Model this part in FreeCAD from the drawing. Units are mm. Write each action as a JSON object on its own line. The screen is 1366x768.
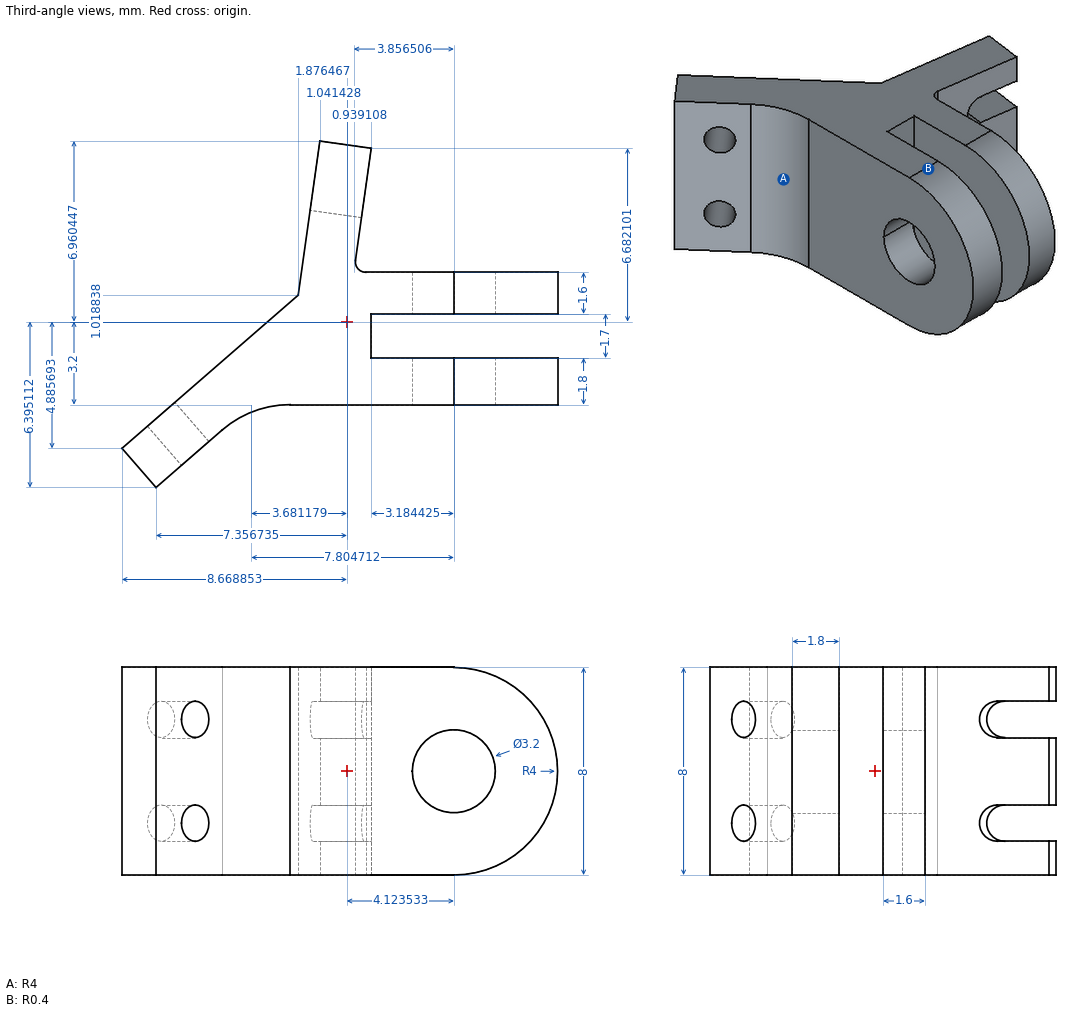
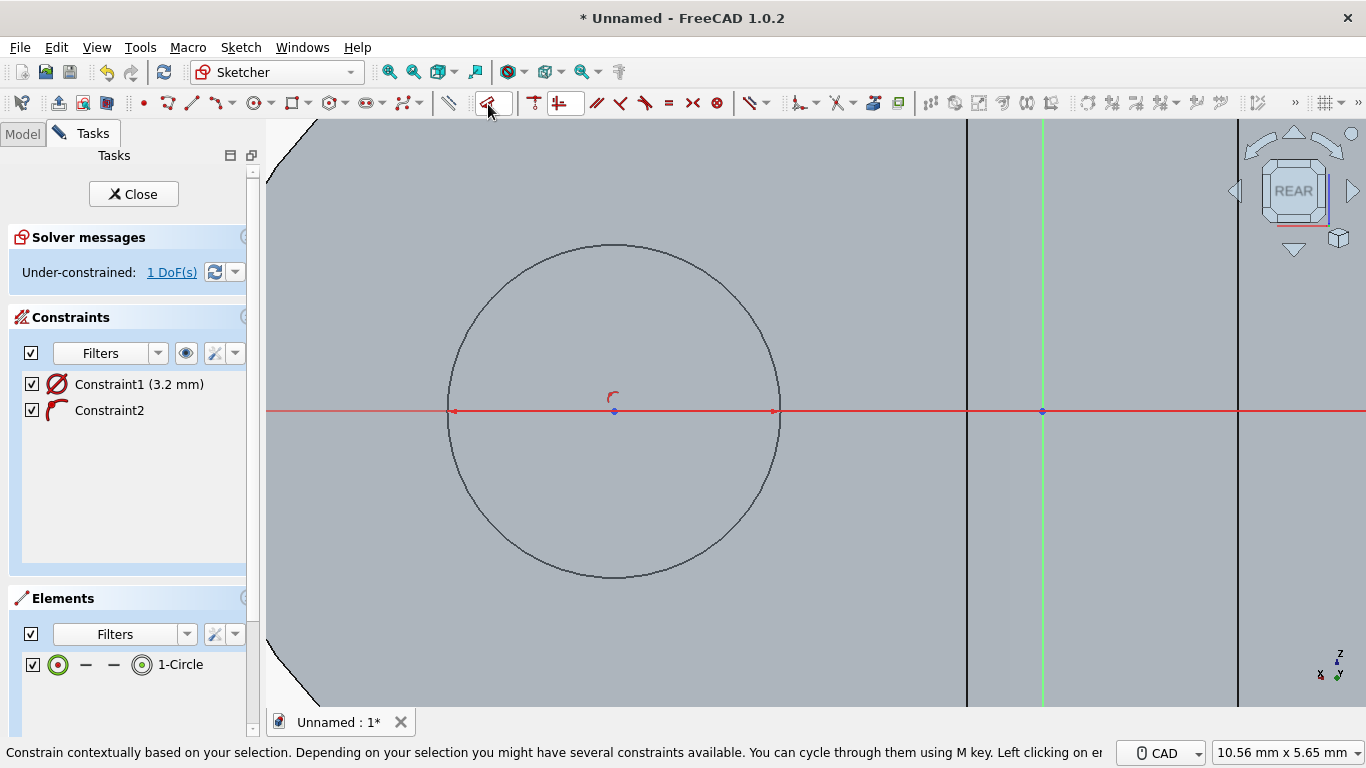
{"action": "left_click", "coordinate": [614, 411]}
{"action": "left_click", "coordinate": [828, 445]}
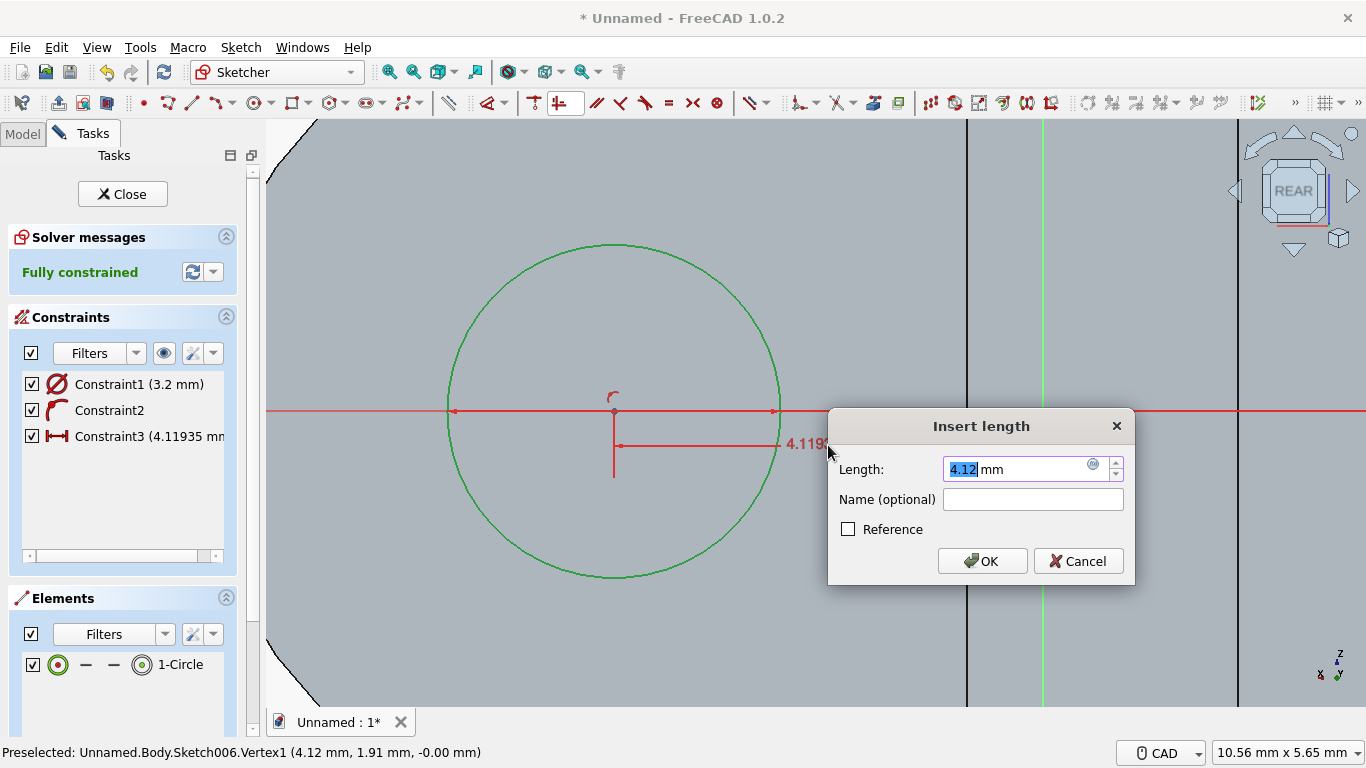
{"action": "type", "text": "4.123533"}
{"action": "key", "text": "Return"}
{"action": "key", "text": "Escape"}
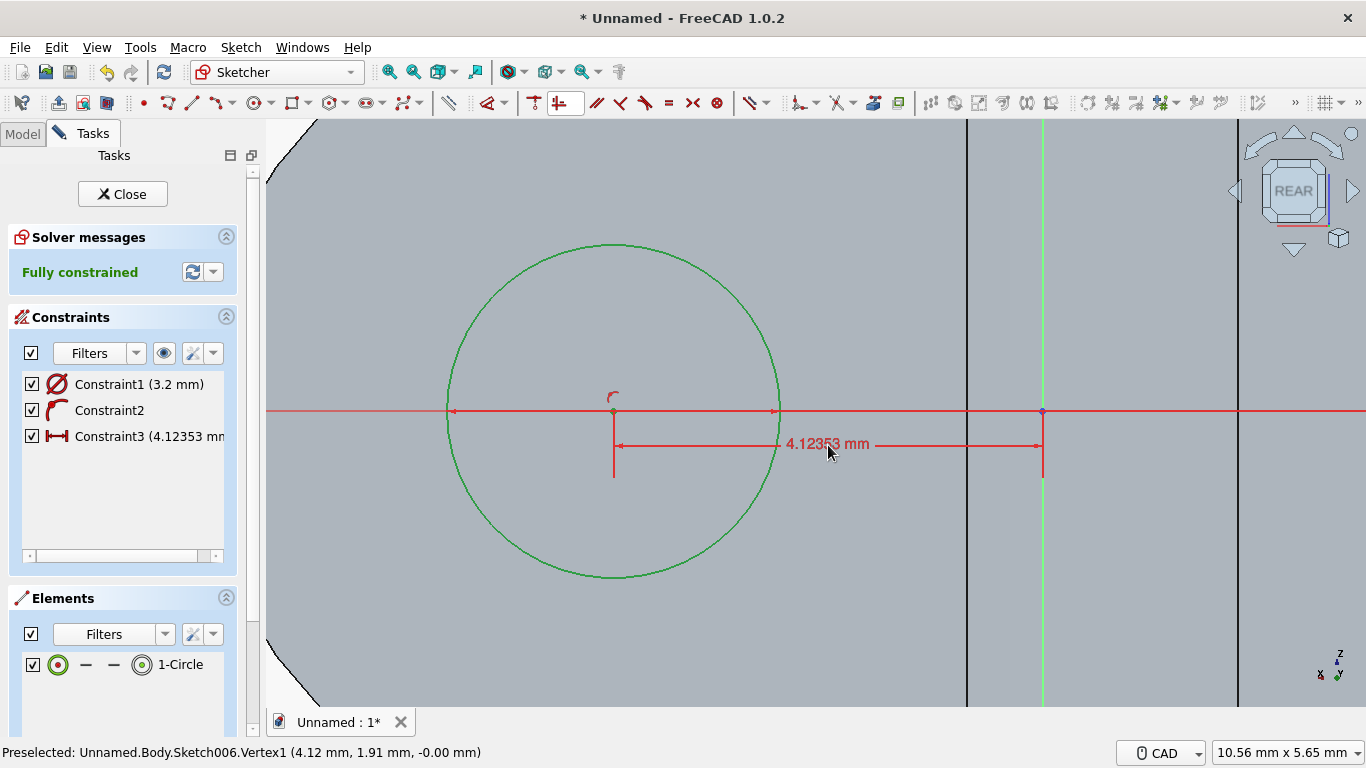
{"action": "left_click", "coordinate": [123, 194]}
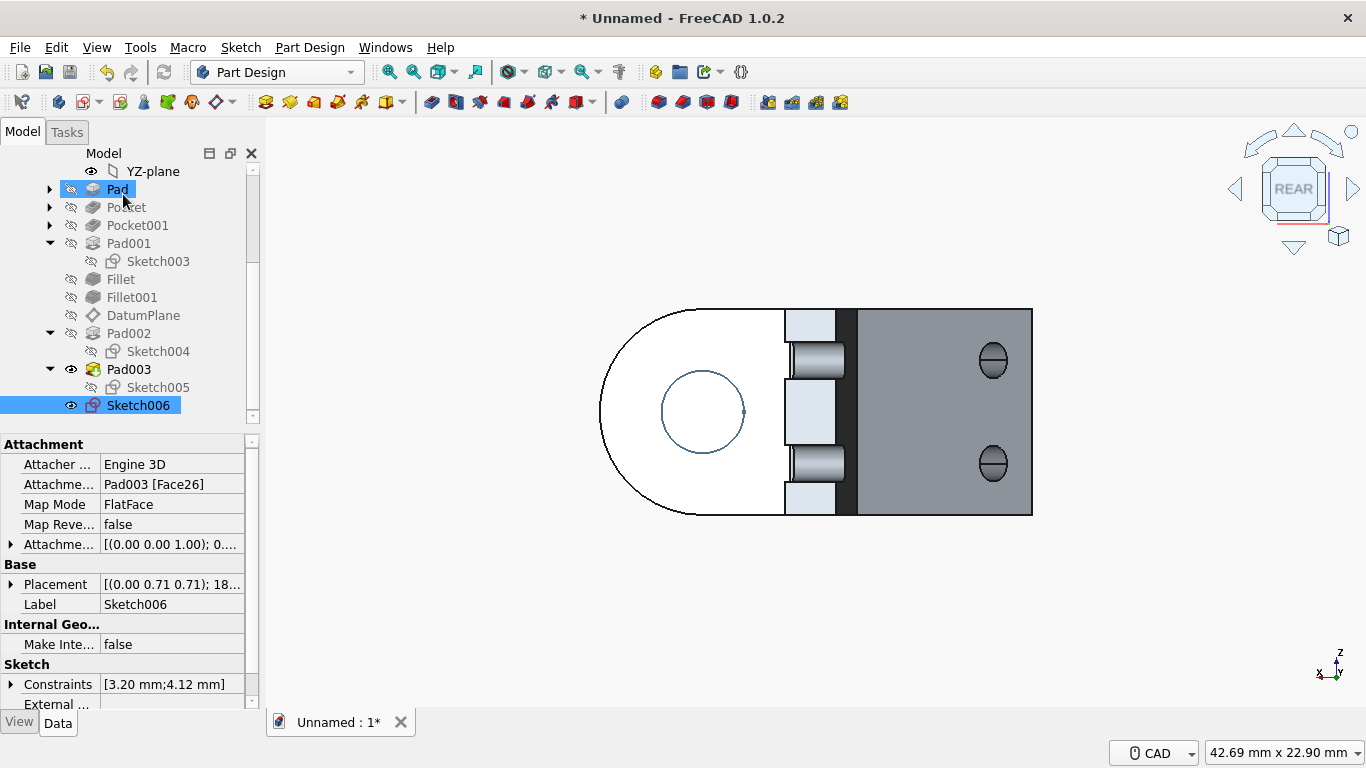
{"action": "left_click", "coordinate": [432, 102]}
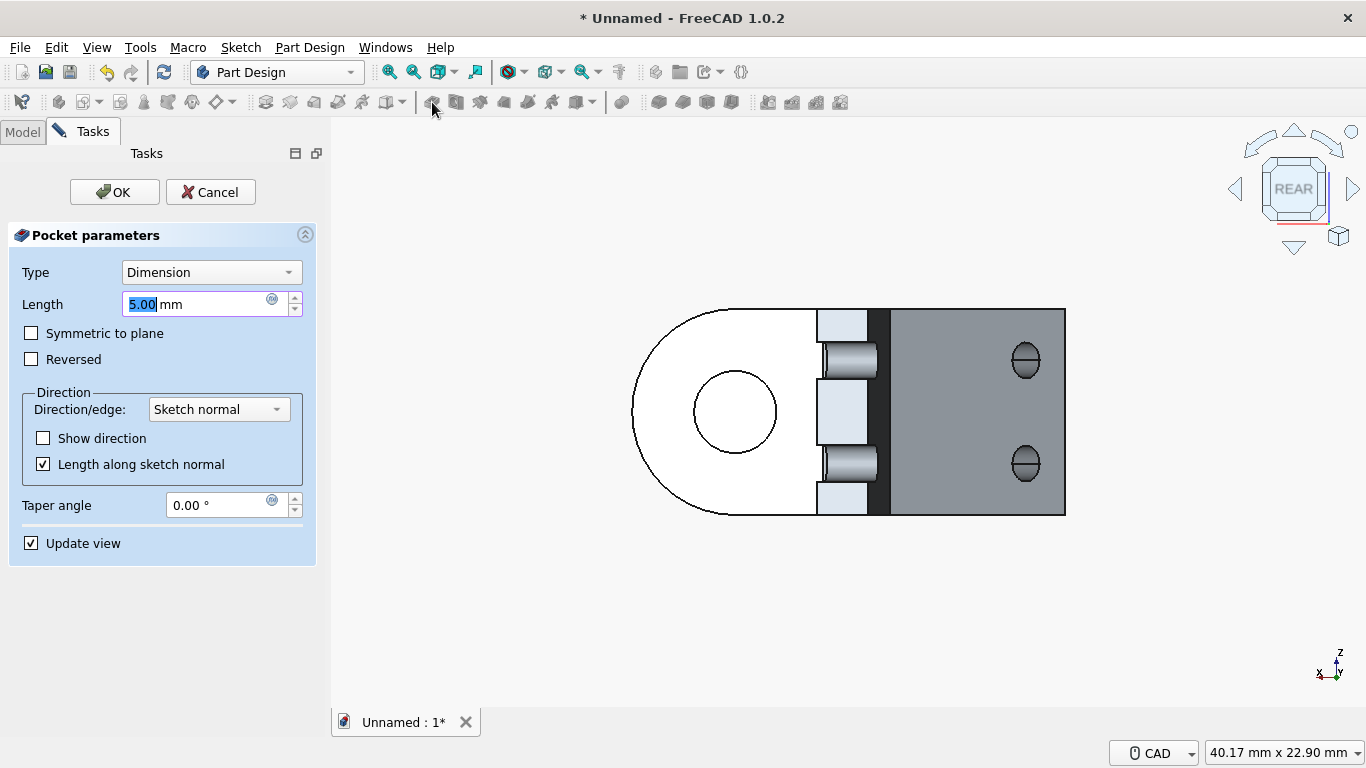
{"action": "left_click", "coordinate": [212, 272]}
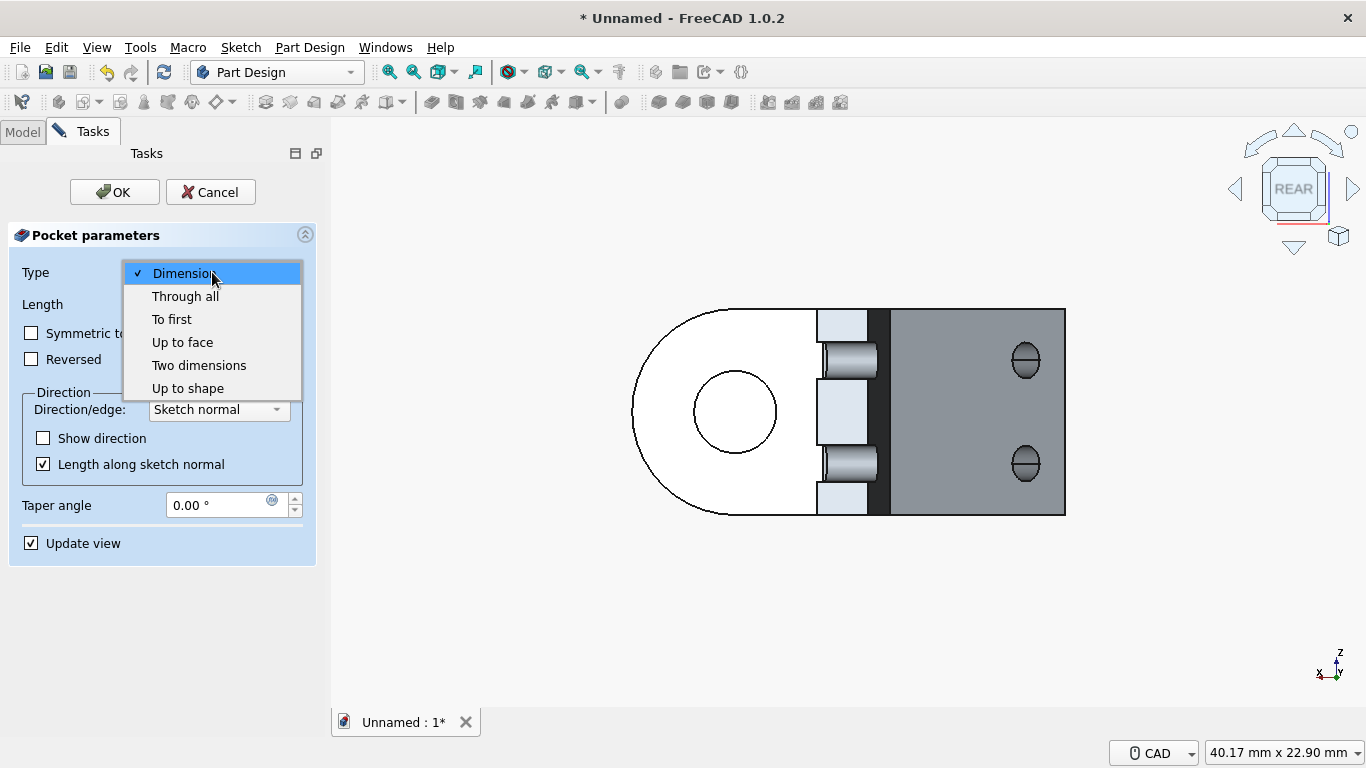
{"action": "left_click", "coordinate": [212, 296]}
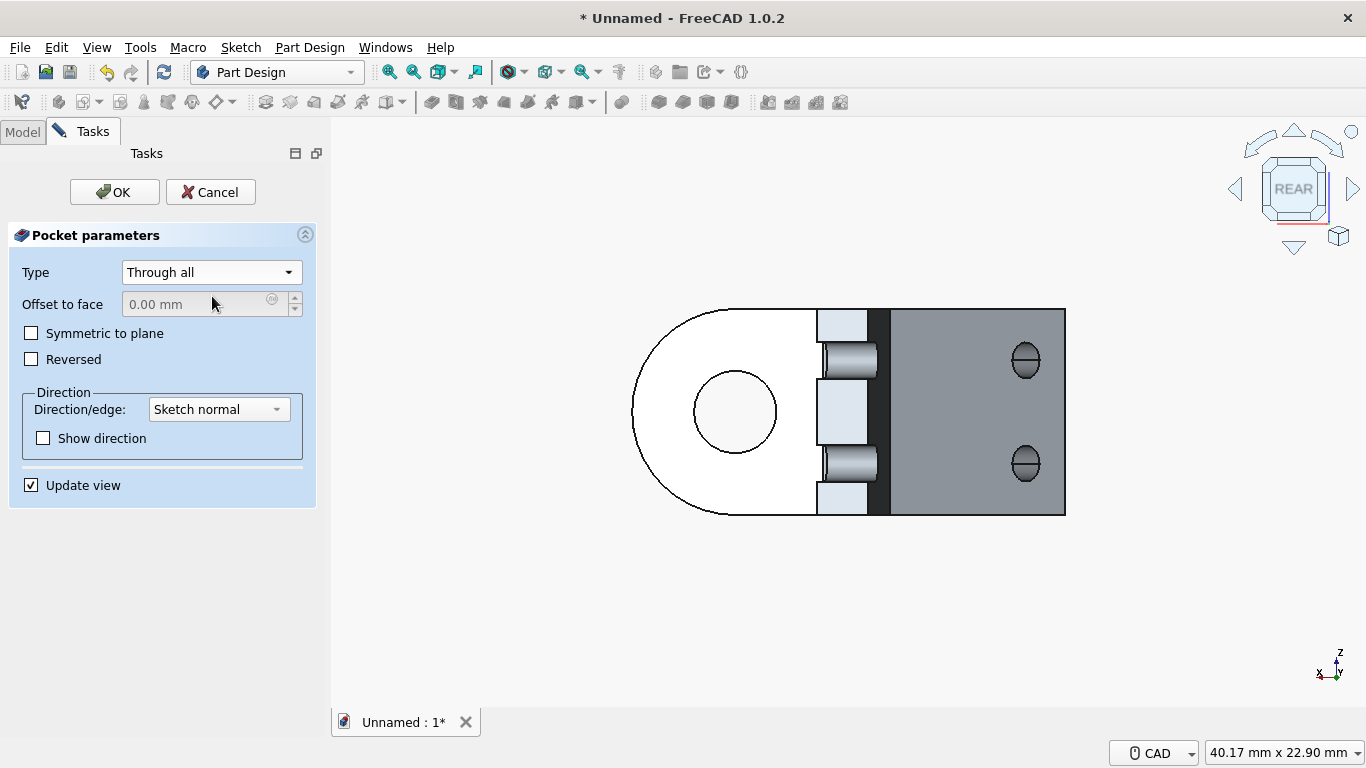
{"action": "left_click", "coordinate": [115, 192]}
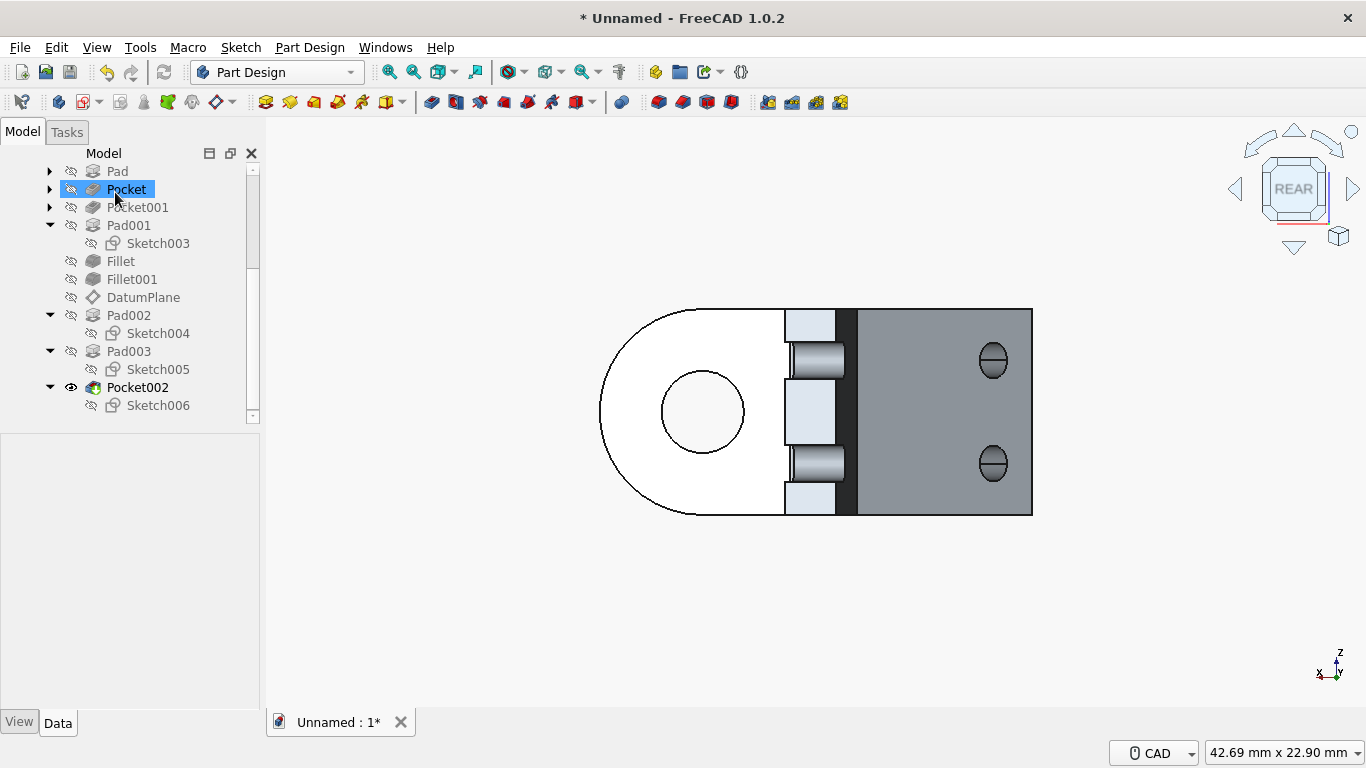
{"action": "key", "text": "0"}